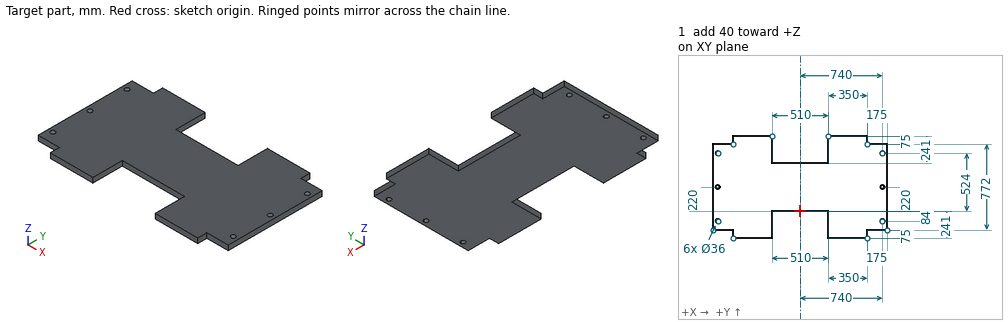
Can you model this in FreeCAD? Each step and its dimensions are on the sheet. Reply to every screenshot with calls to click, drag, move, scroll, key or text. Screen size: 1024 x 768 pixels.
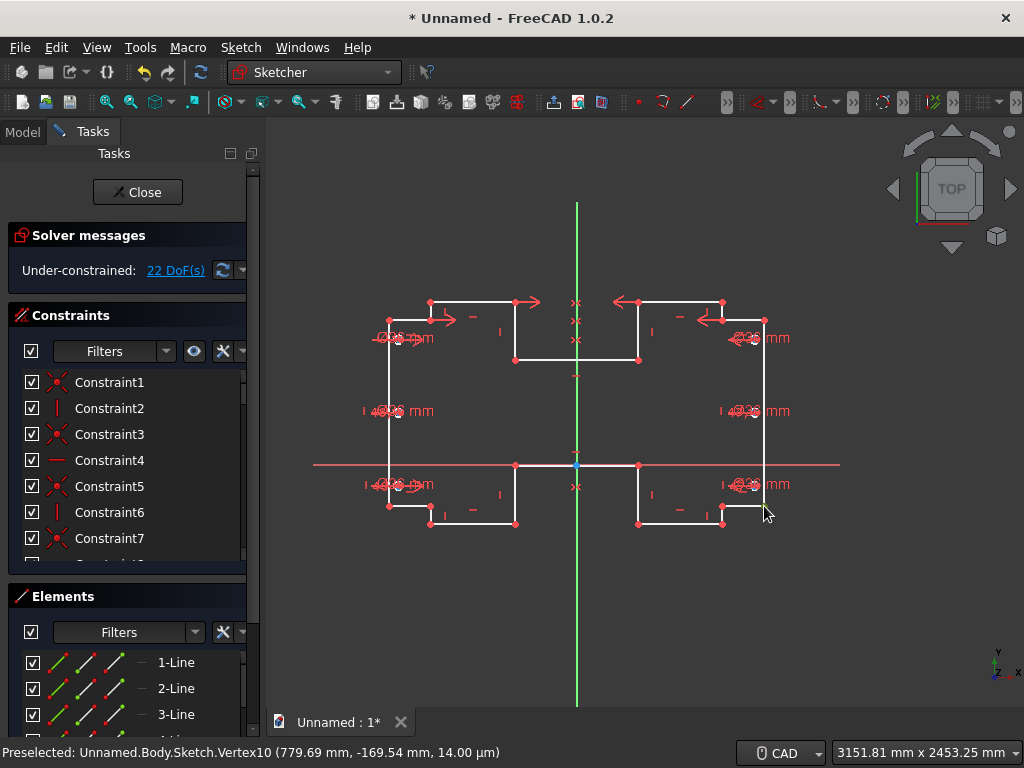
click(389, 506)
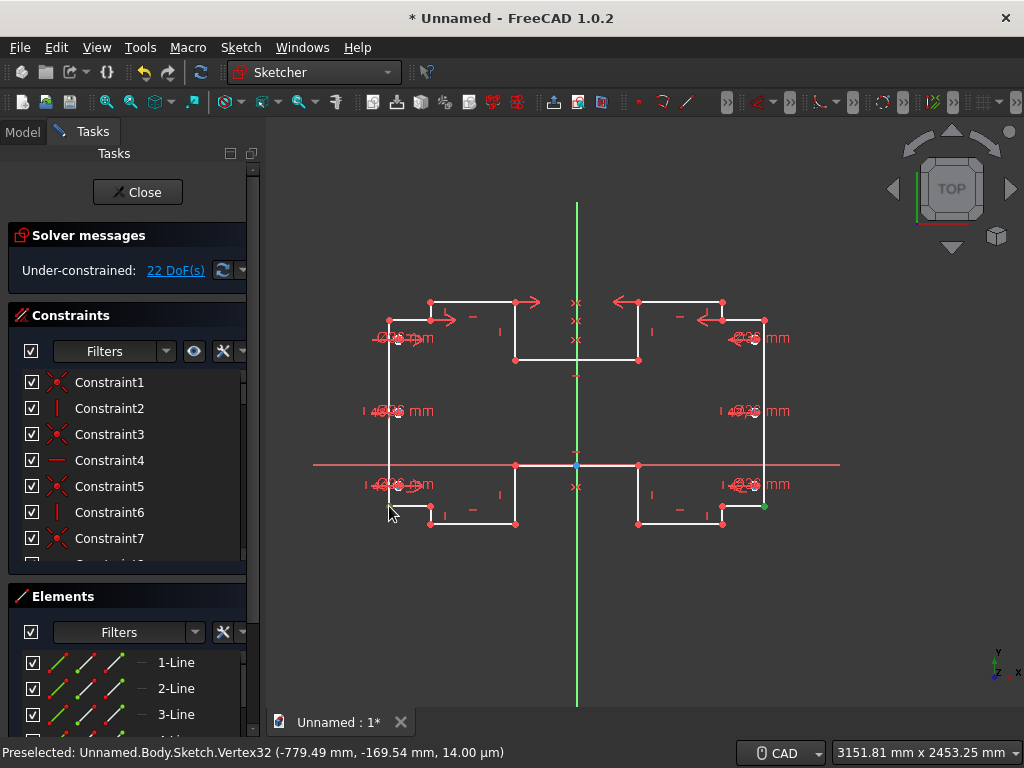
click(577, 641)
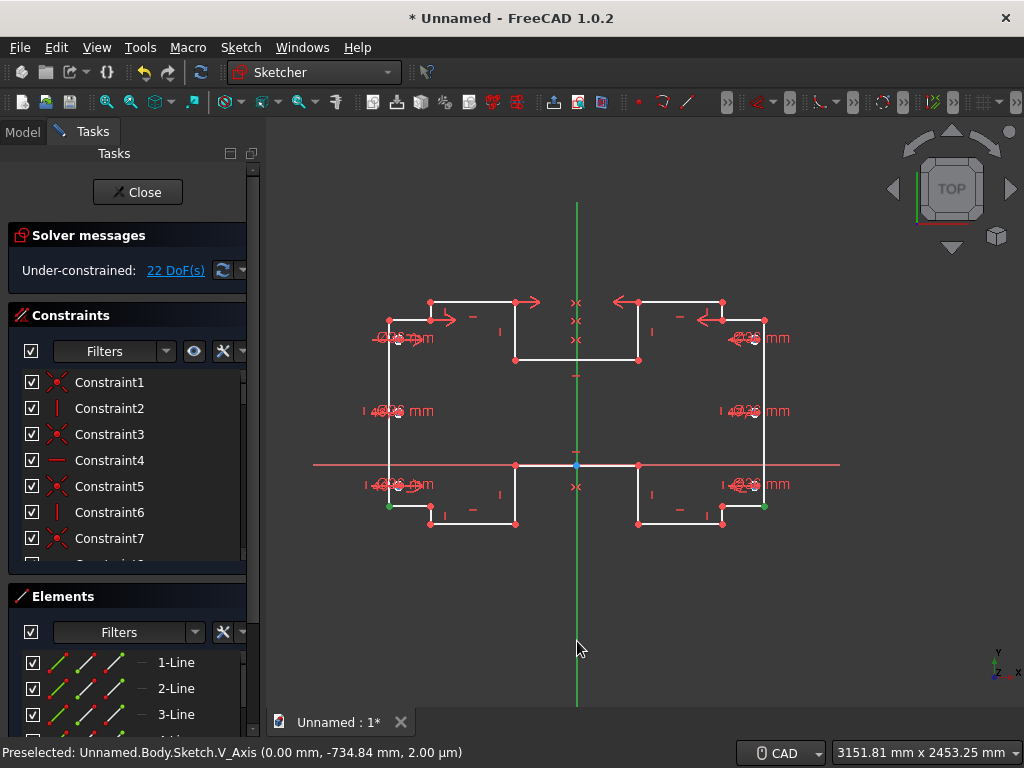
key(s)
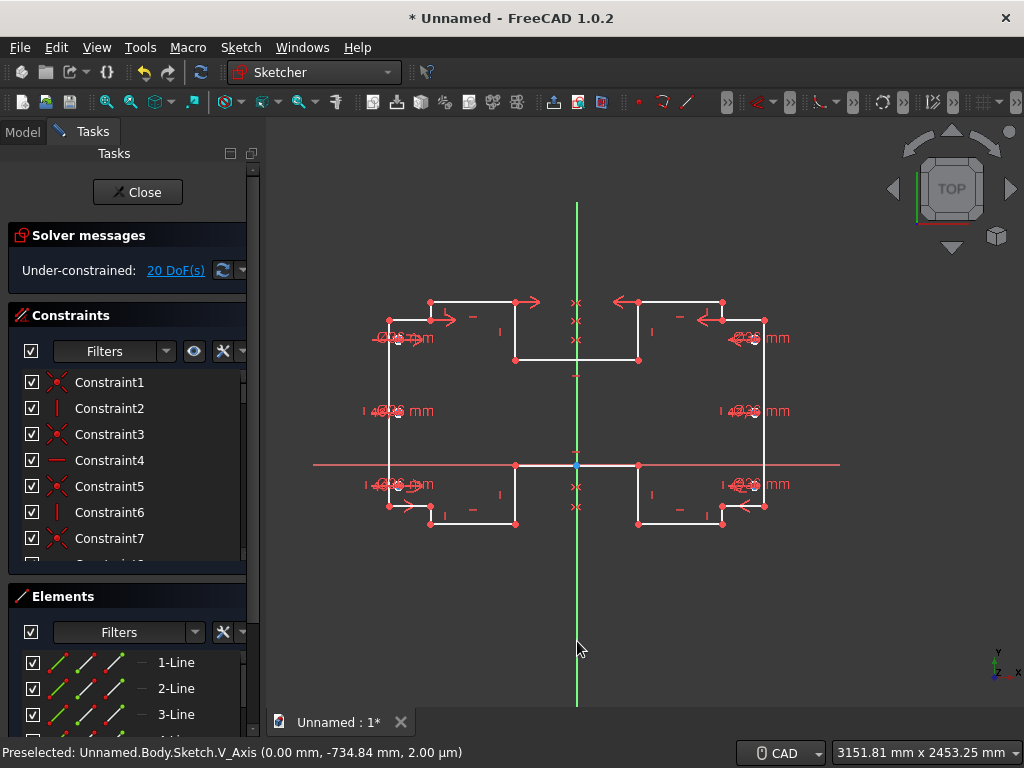
click(722, 524)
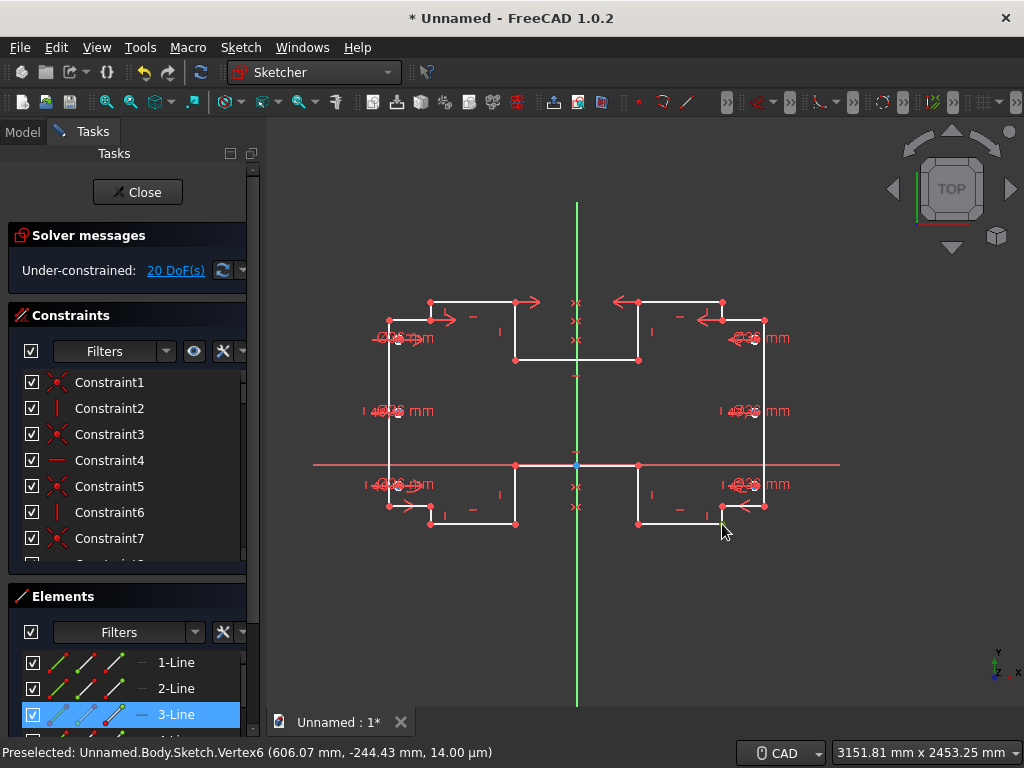
click(431, 524)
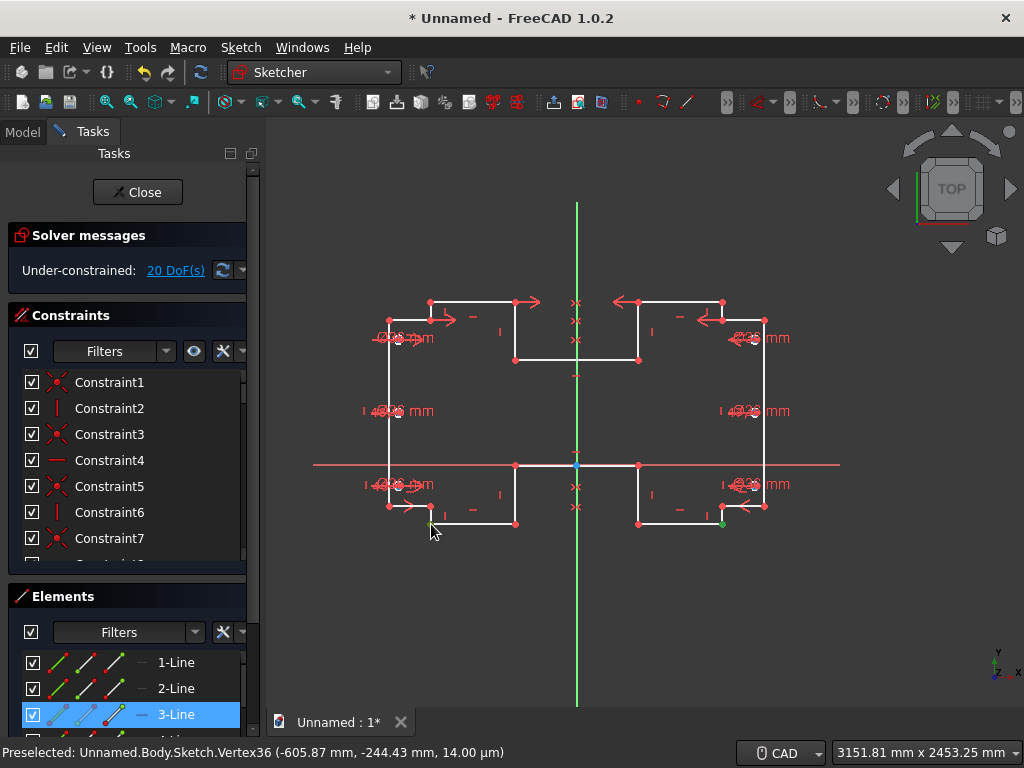
click(577, 641)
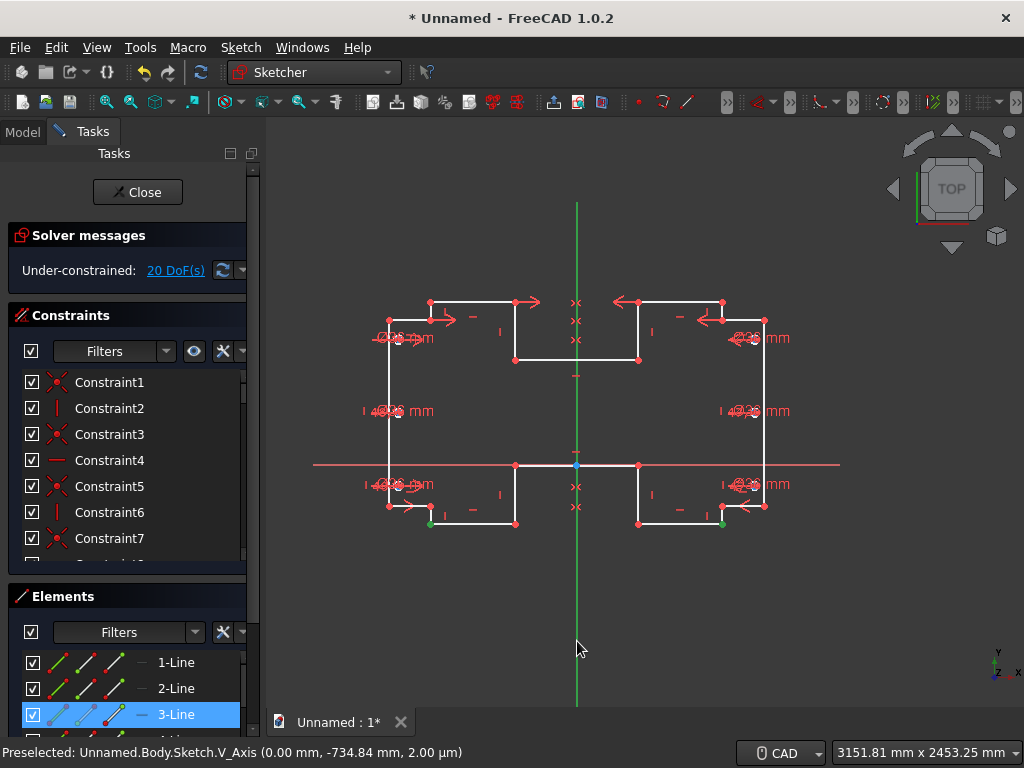
key(s)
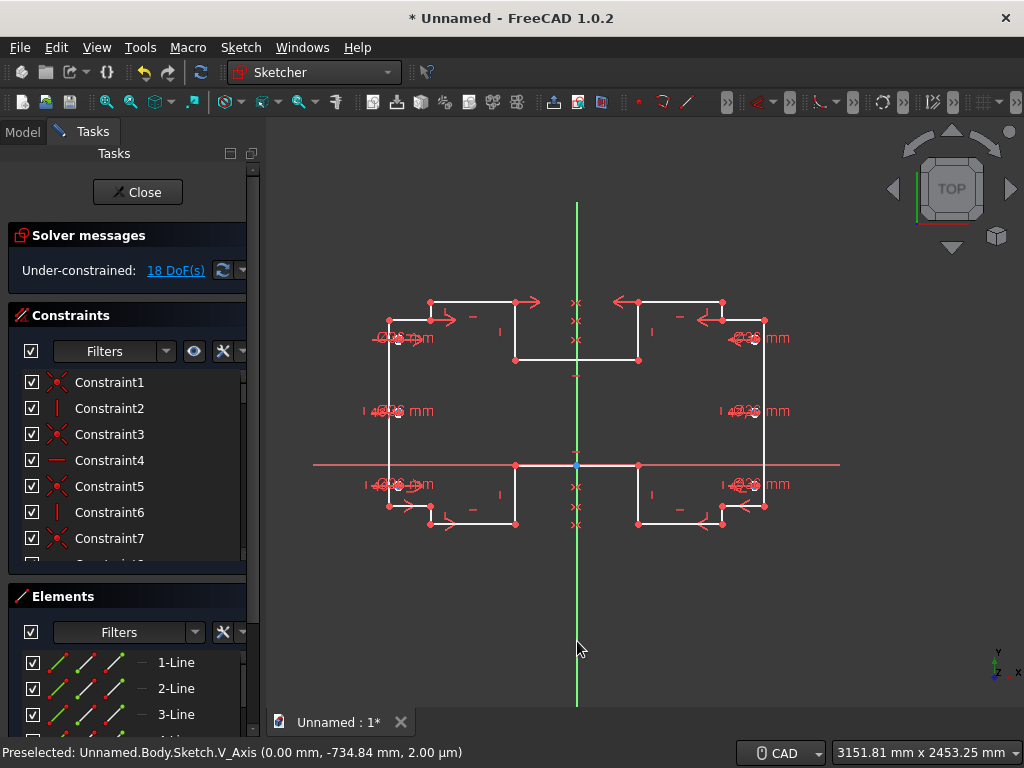
click(515, 466)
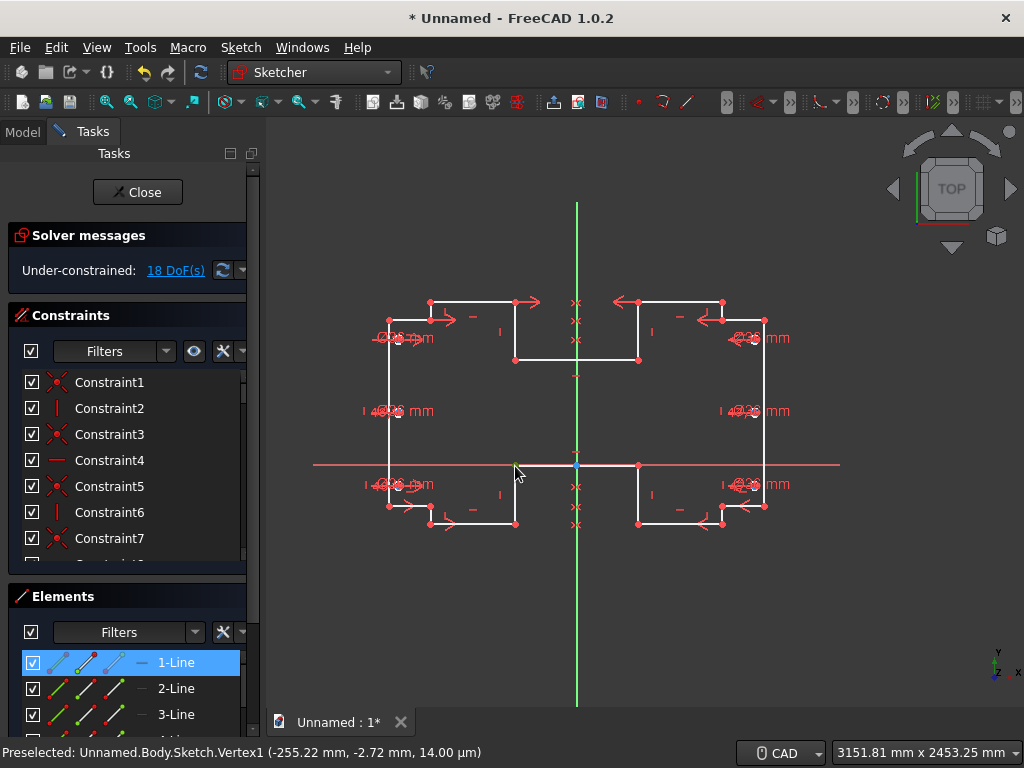
click(334, 465)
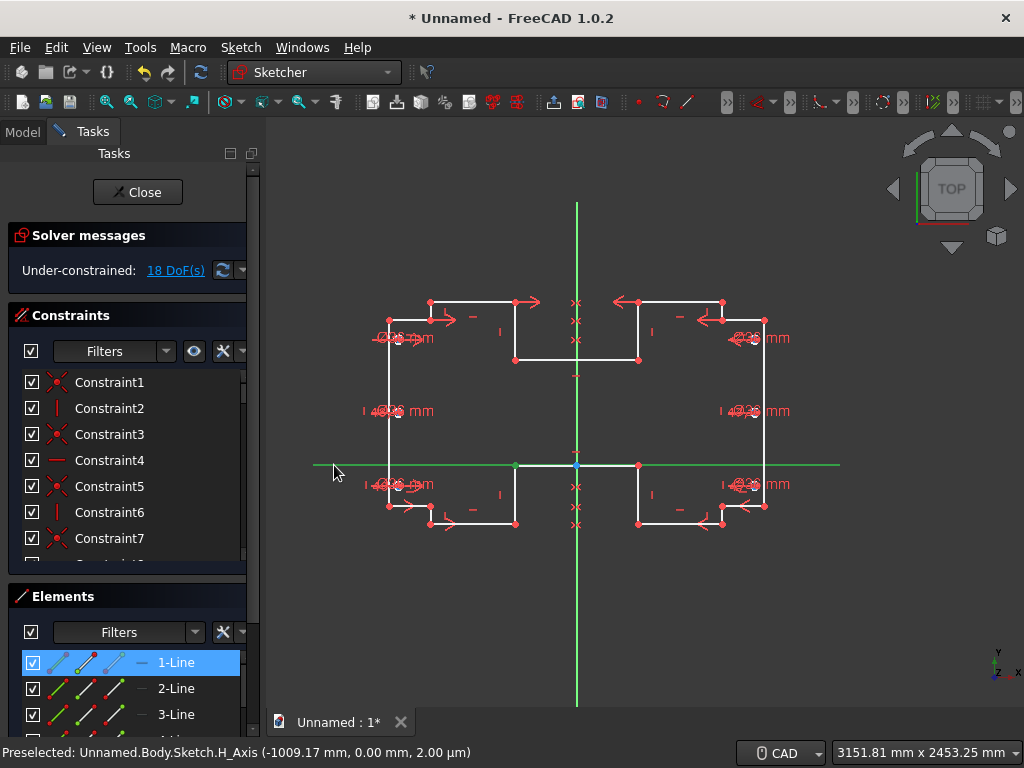
key(c)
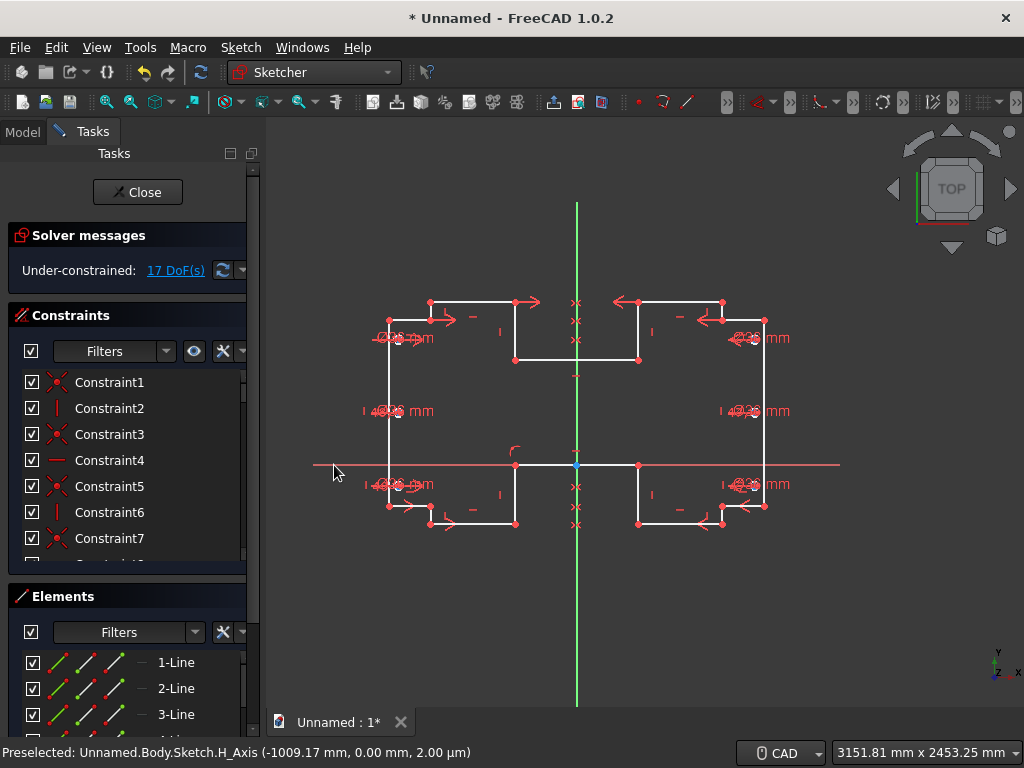
click(758, 102)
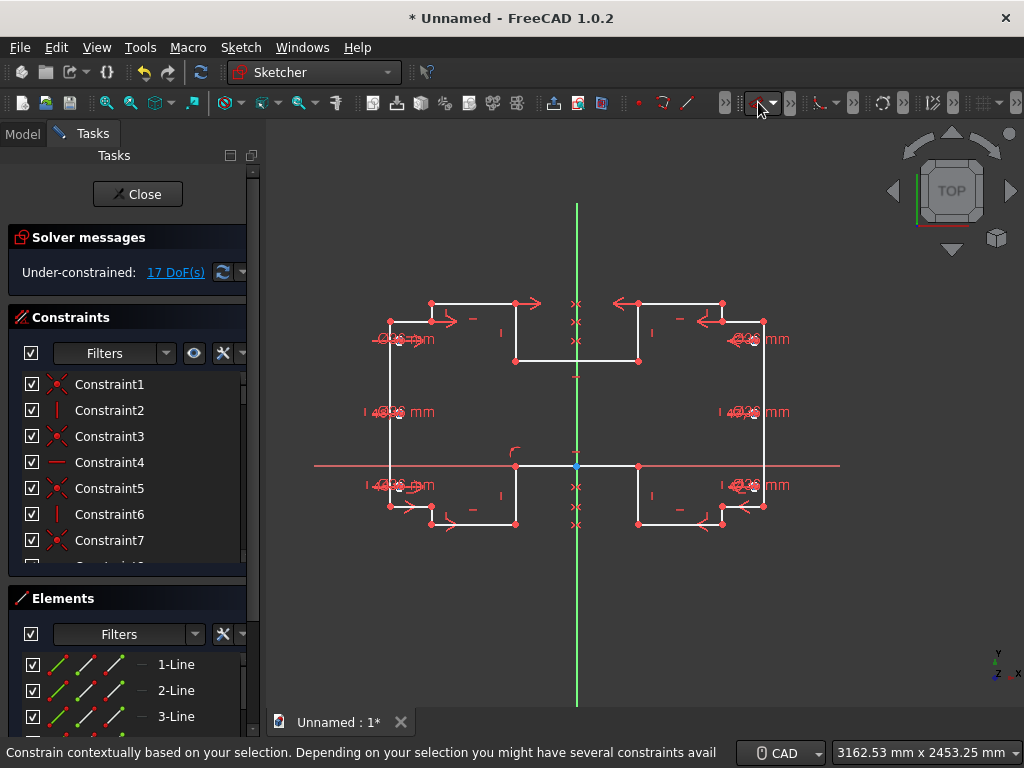
scroll(722, 516, up, 4)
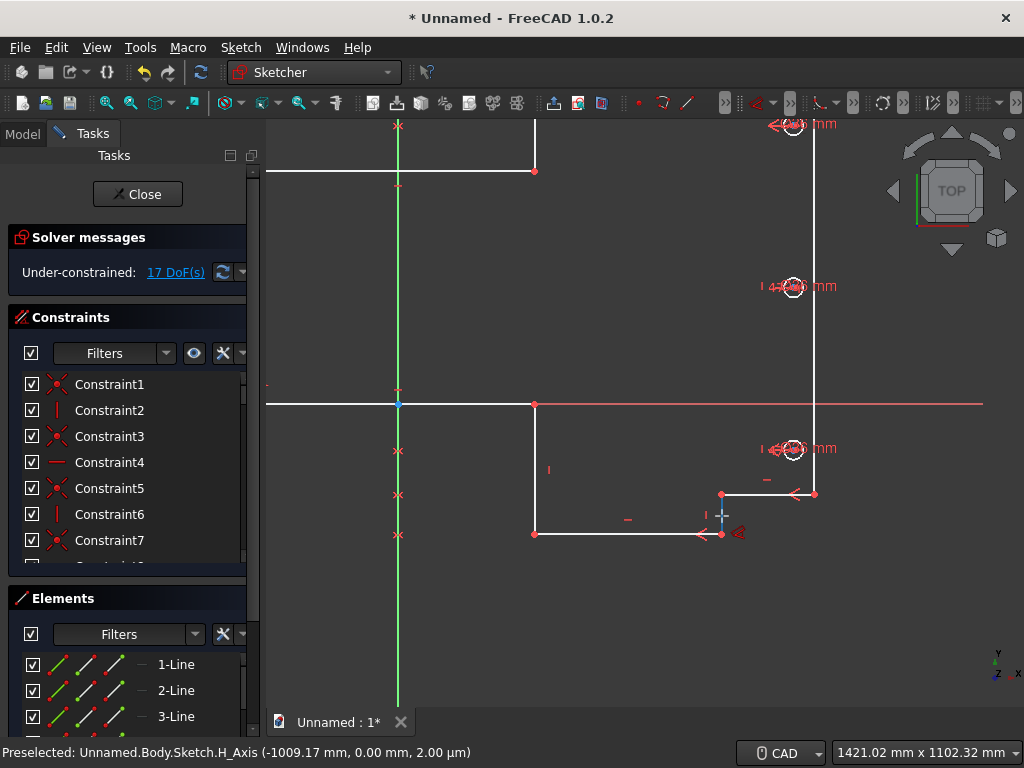
click(722, 515)
click(756, 515)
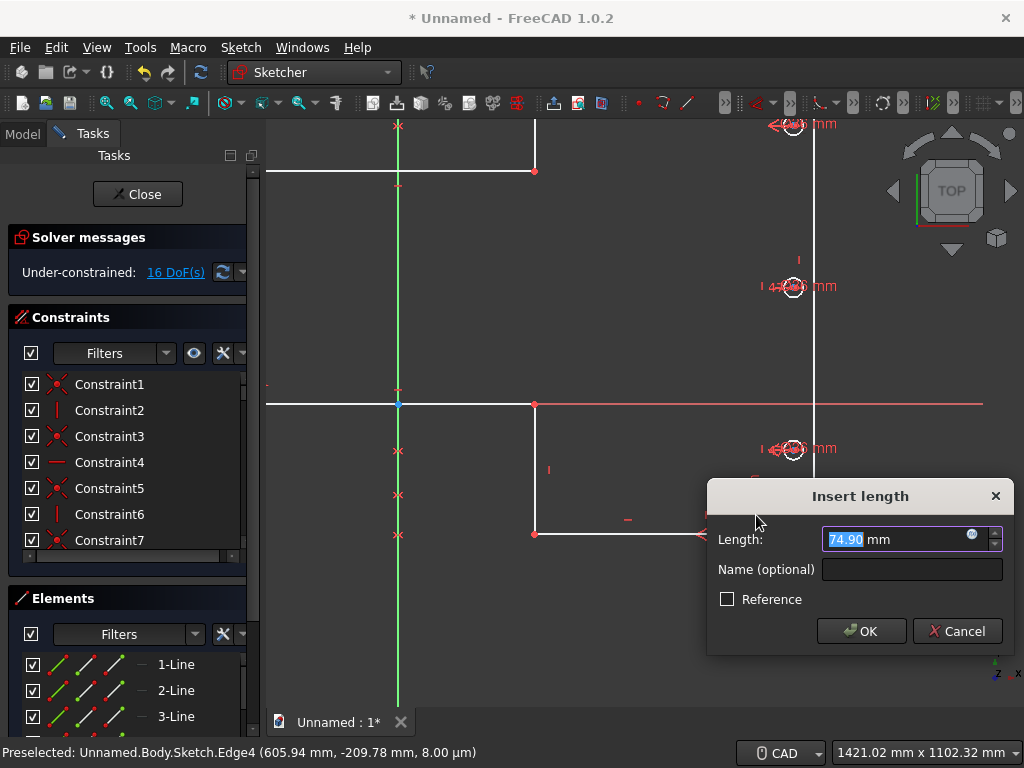
text(75)
key(Return)